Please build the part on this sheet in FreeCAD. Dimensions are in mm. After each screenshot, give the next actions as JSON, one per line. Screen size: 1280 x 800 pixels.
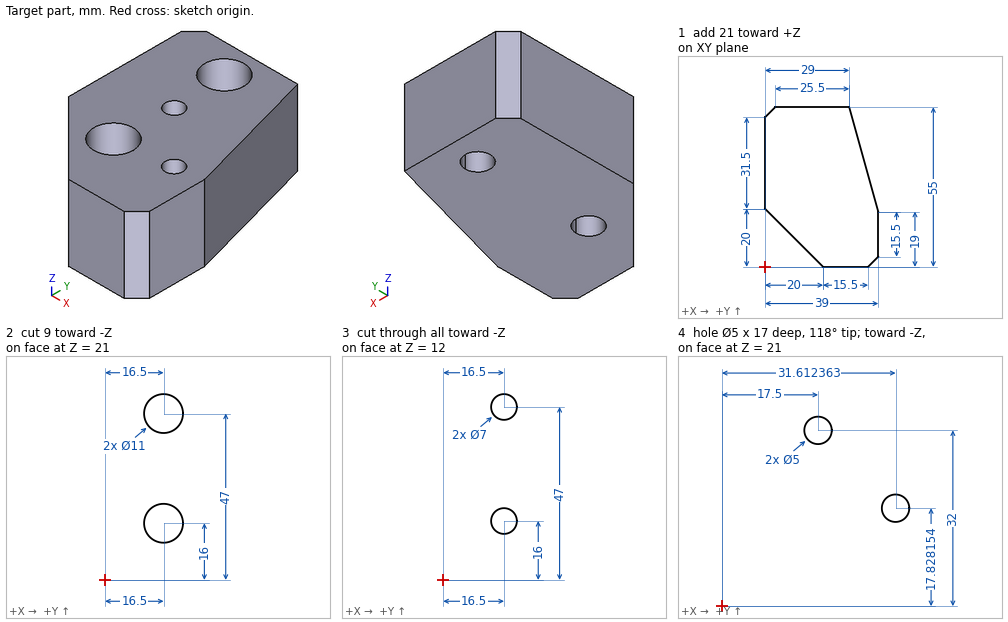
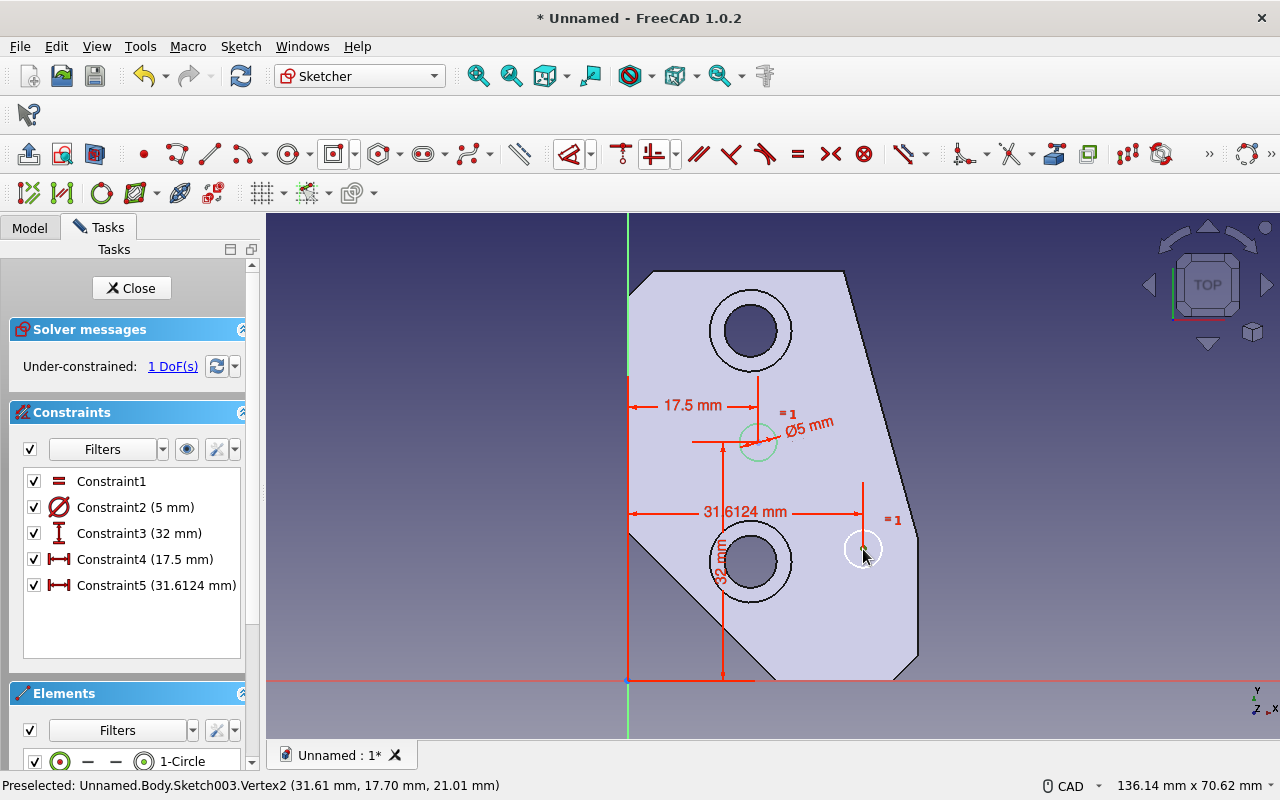
{"action": "left_click", "coordinate": [590, 154]}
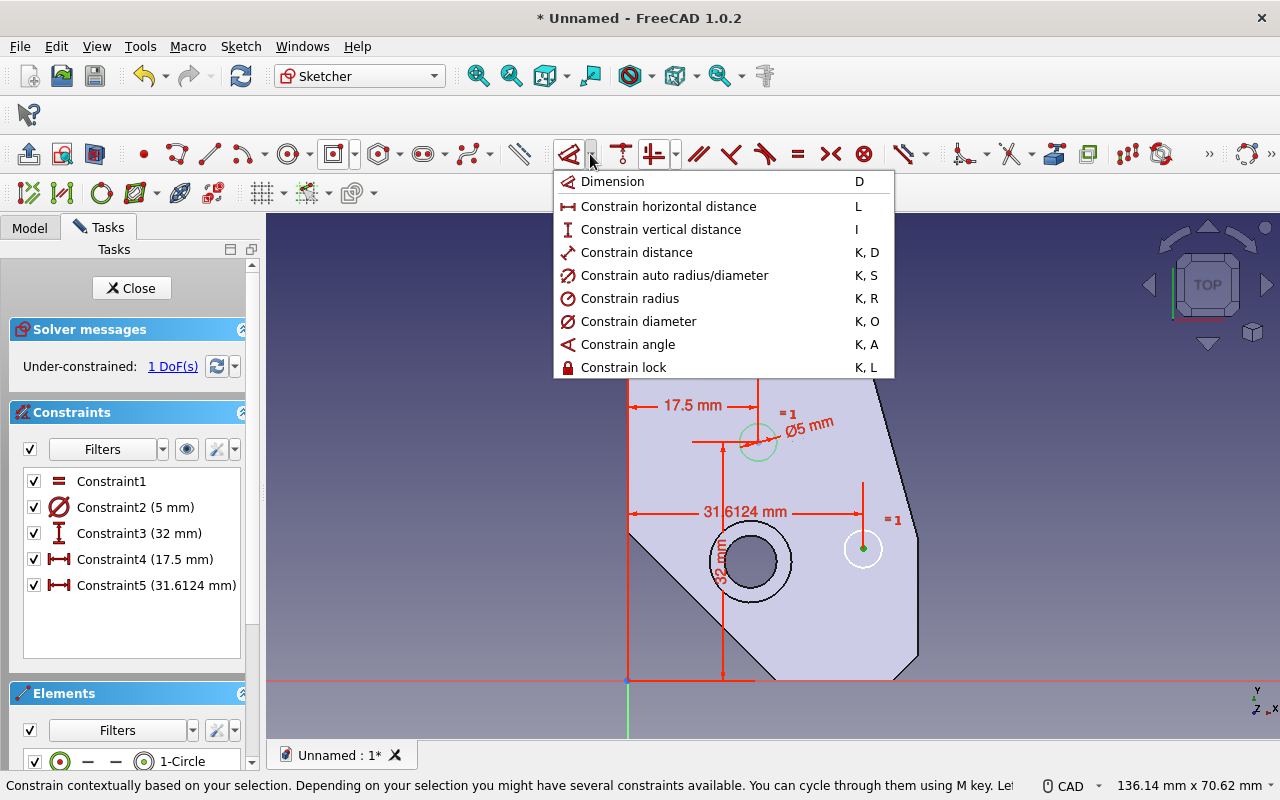
{"action": "left_click", "coordinate": [724, 230]}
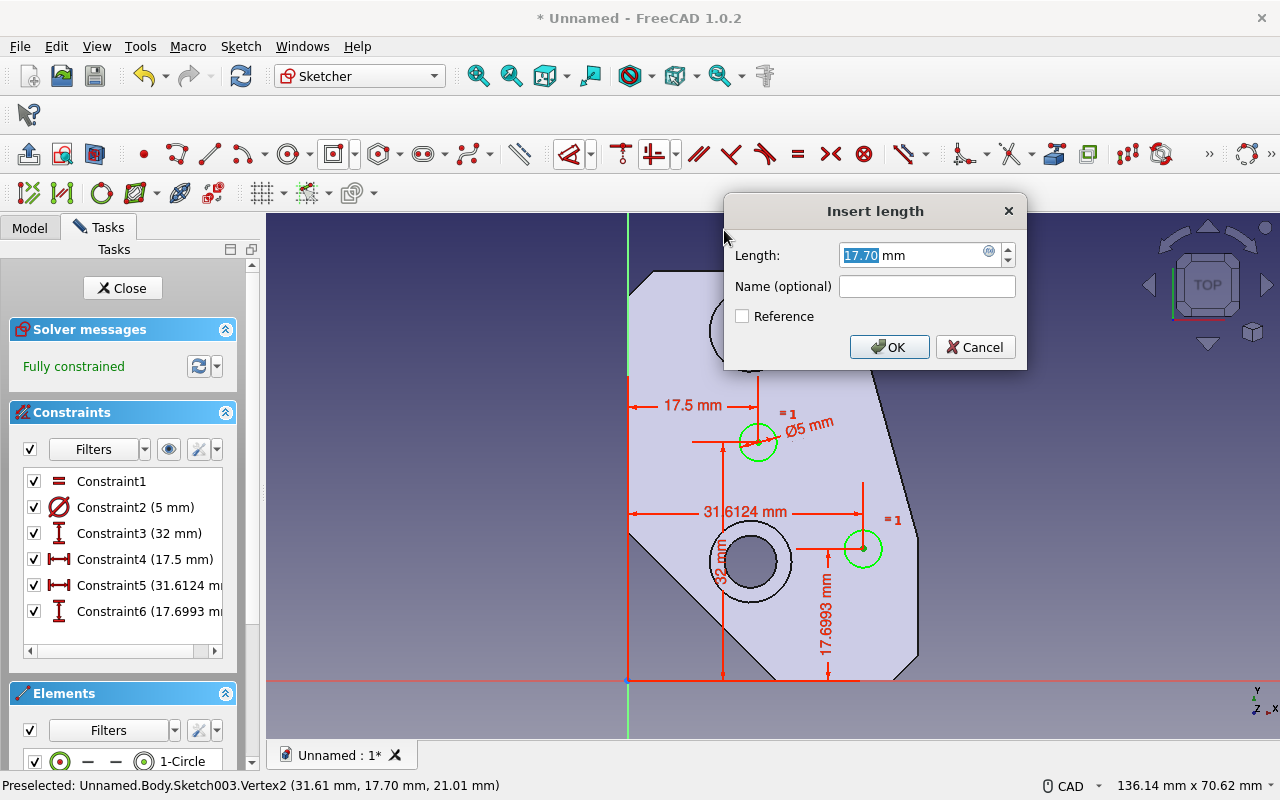
{"action": "type", "text": "17.828154"}
{"action": "key", "text": "Return"}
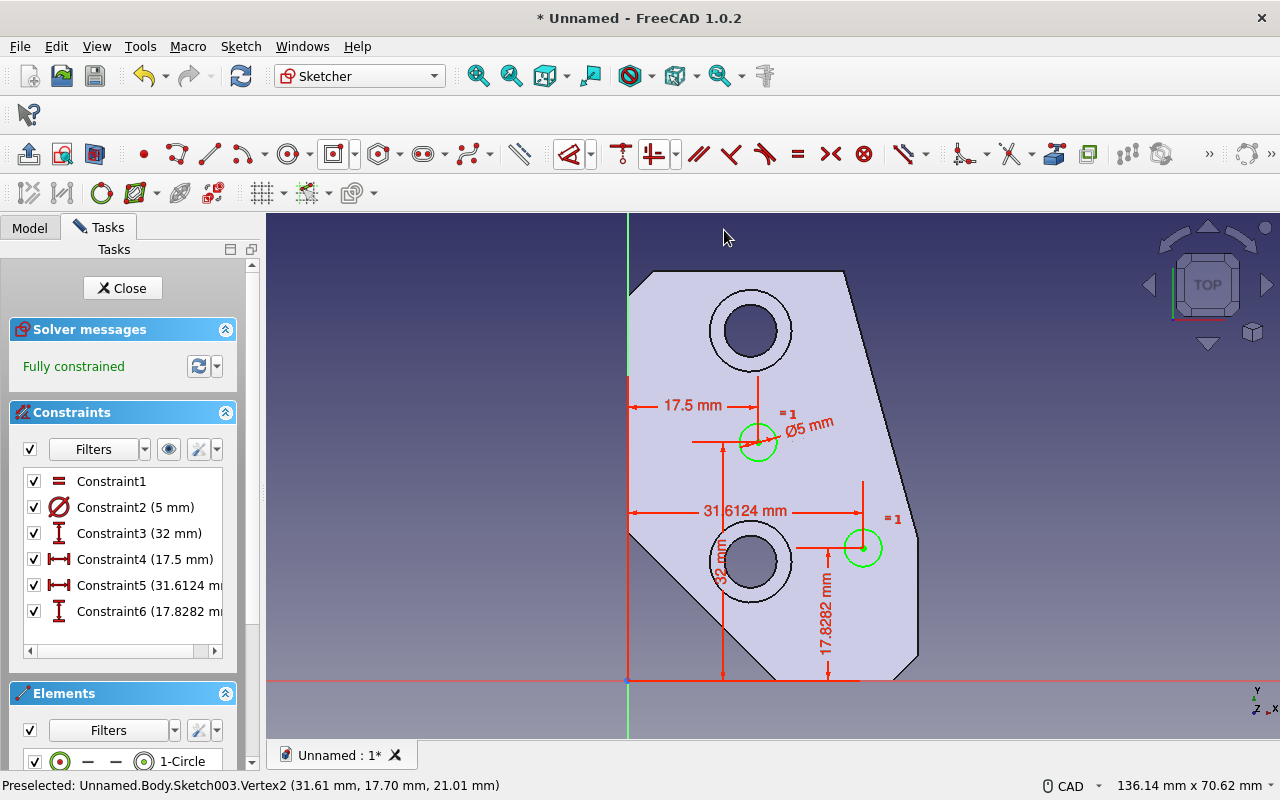
{"action": "left_click", "coordinate": [123, 288]}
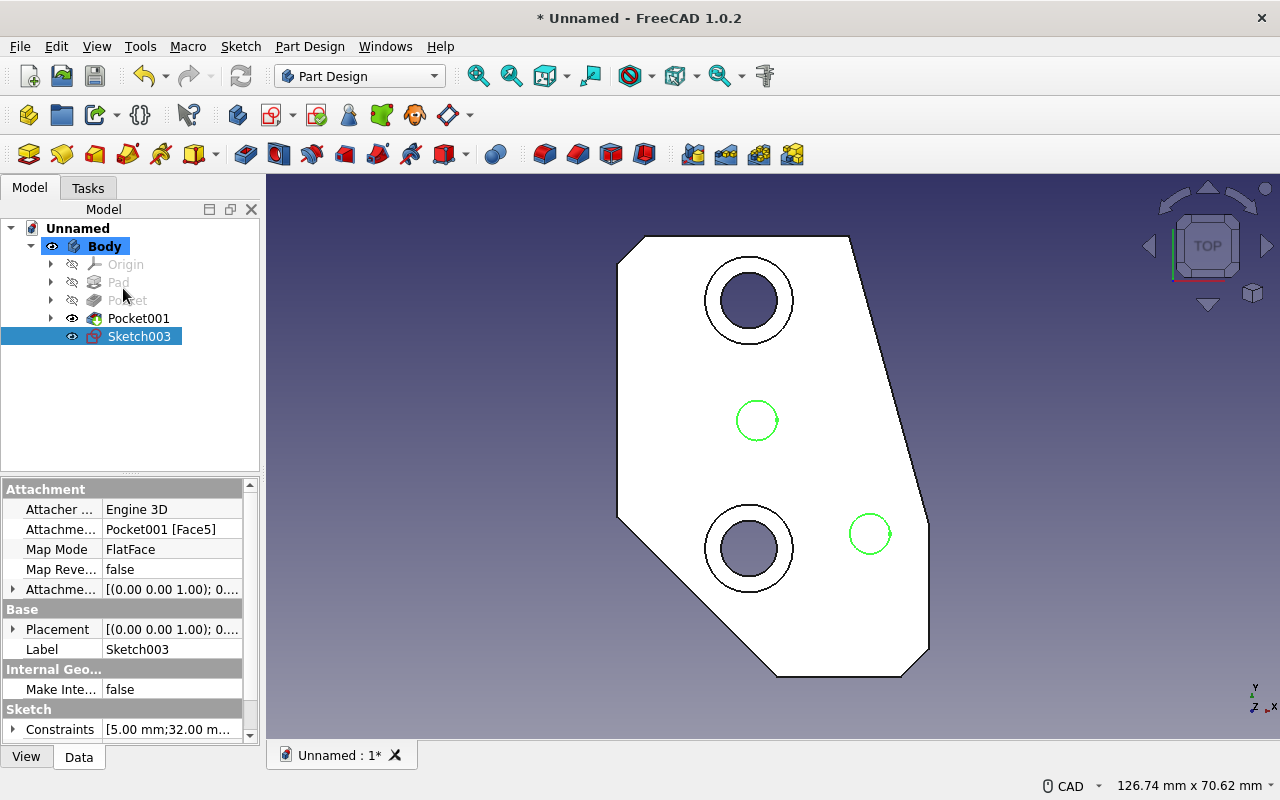
{"action": "left_click", "coordinate": [279, 154]}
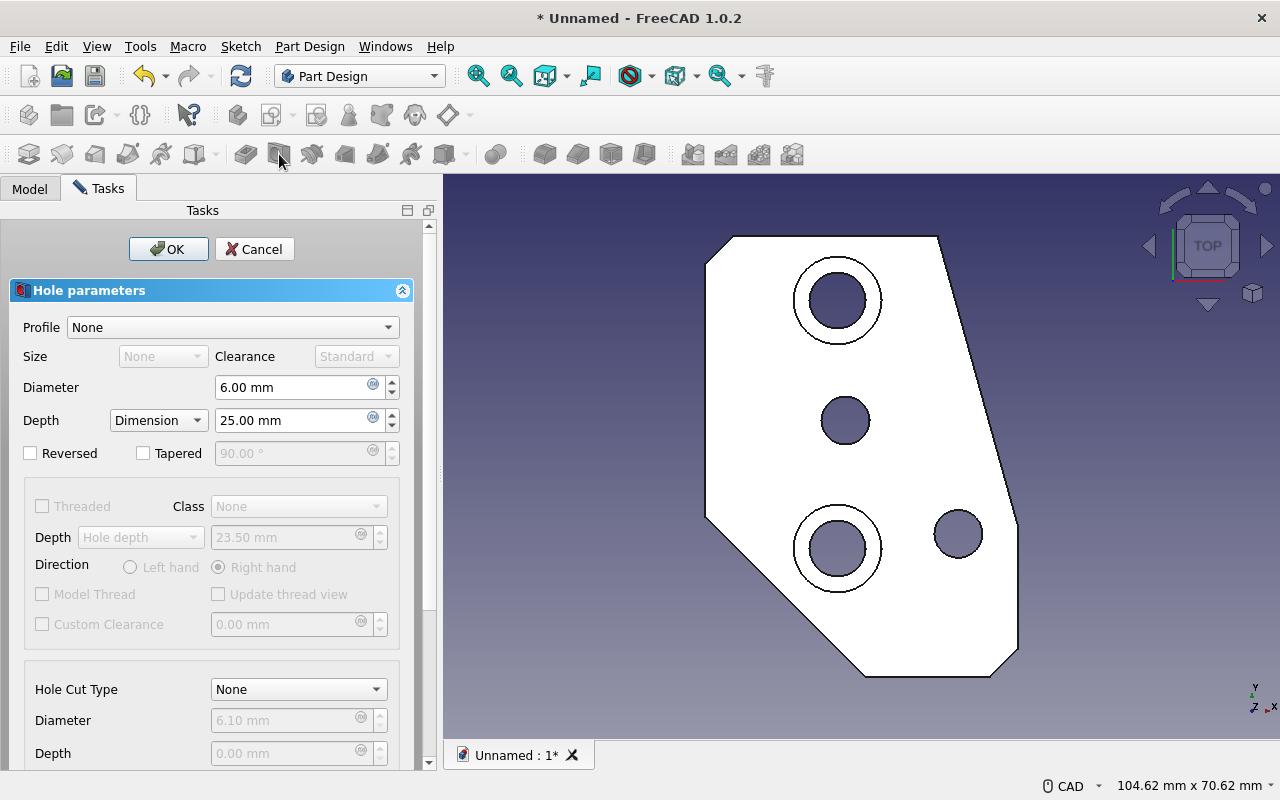
{"action": "triple_click", "coordinate": [300, 388]}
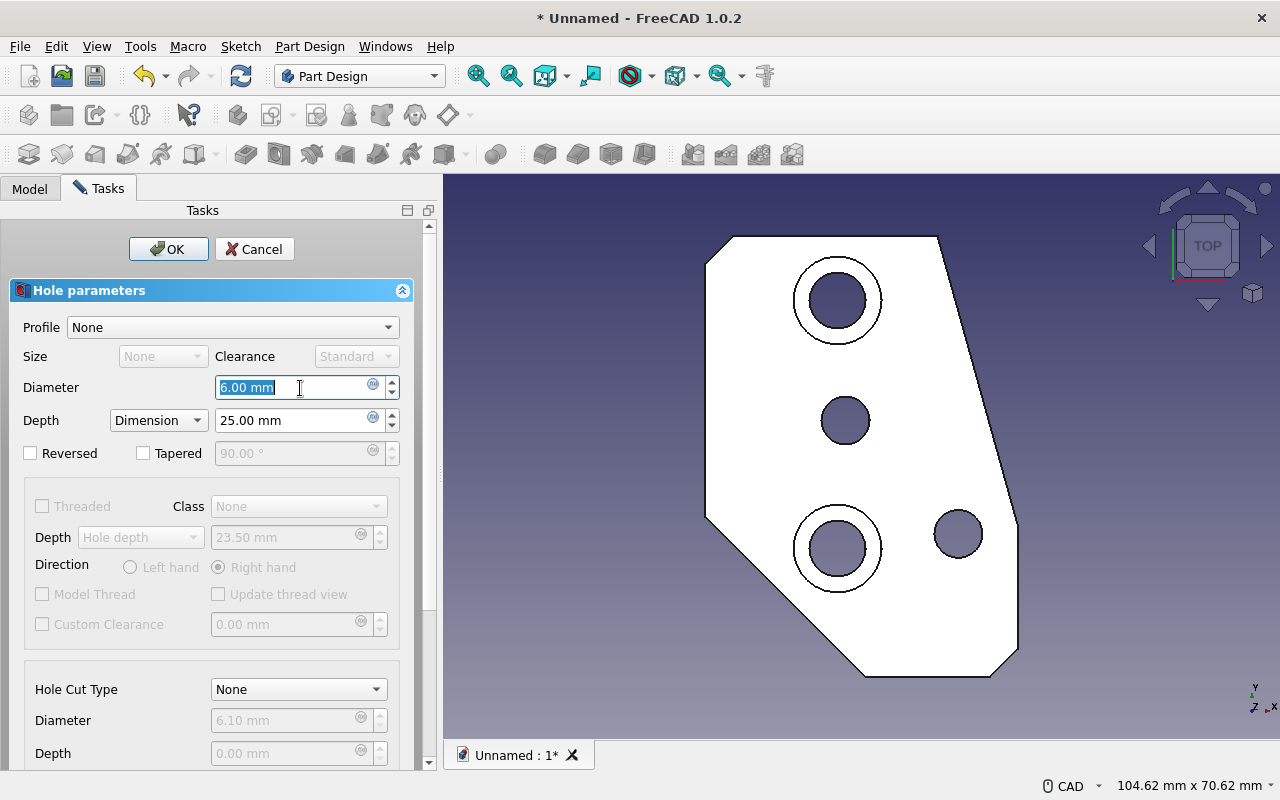
{"action": "type", "text": "5"}
{"action": "key", "text": "Tab"}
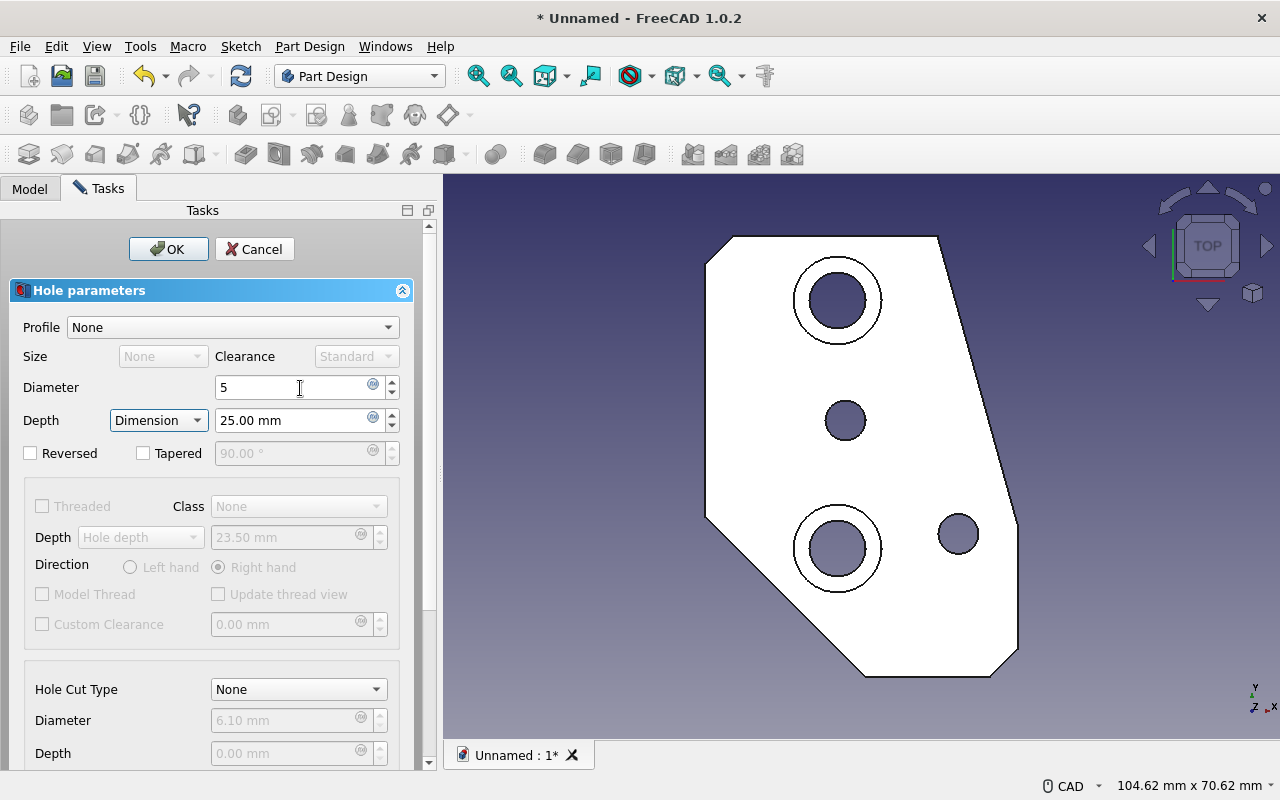
{"action": "triple_click", "coordinate": [300, 420]}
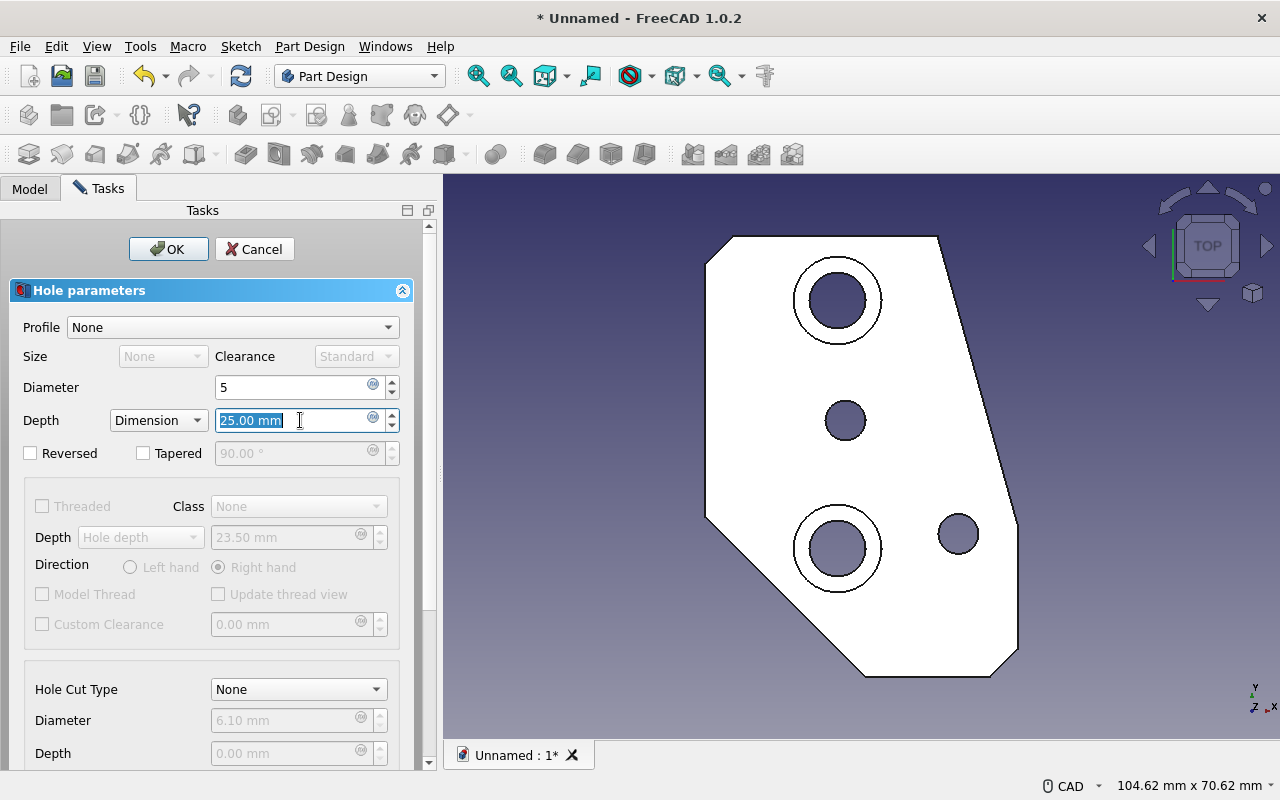
{"action": "type", "text": "17"}
{"action": "key", "text": "Tab"}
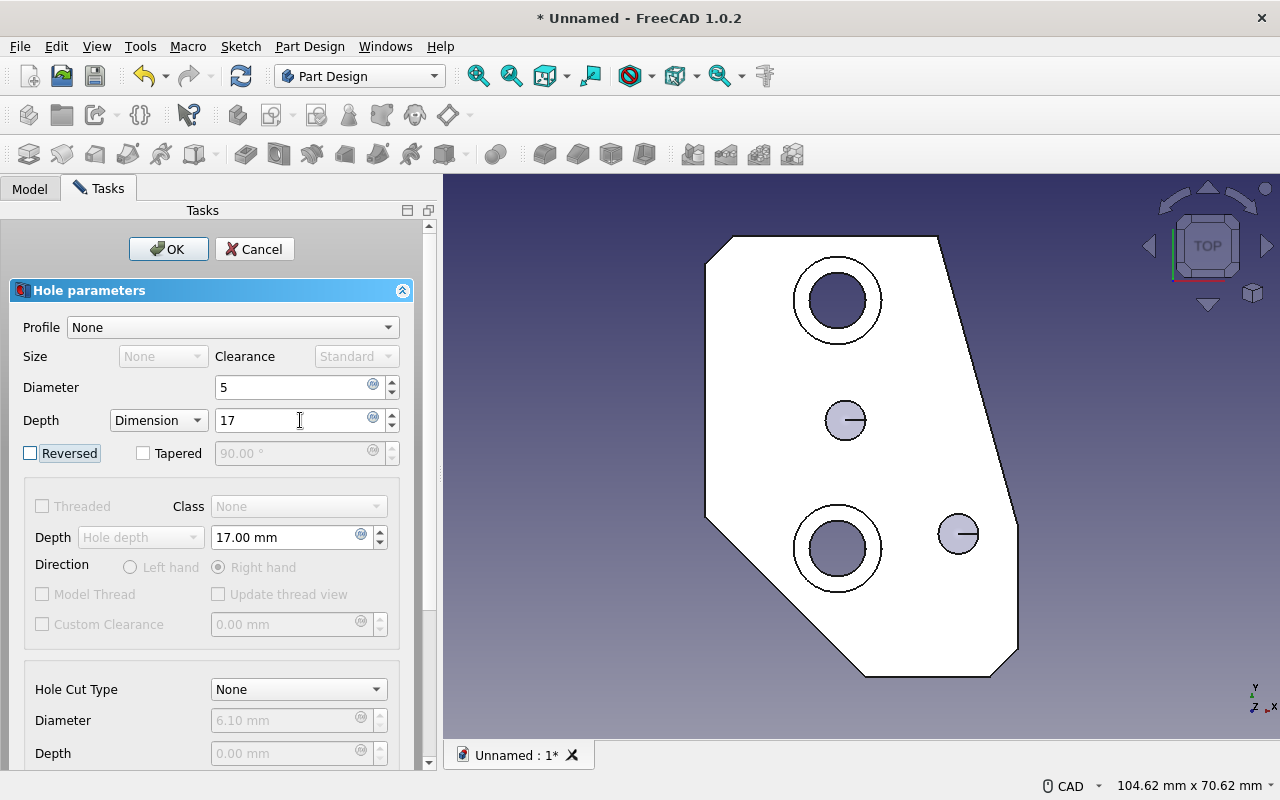
{"action": "left_click", "coordinate": [169, 249]}